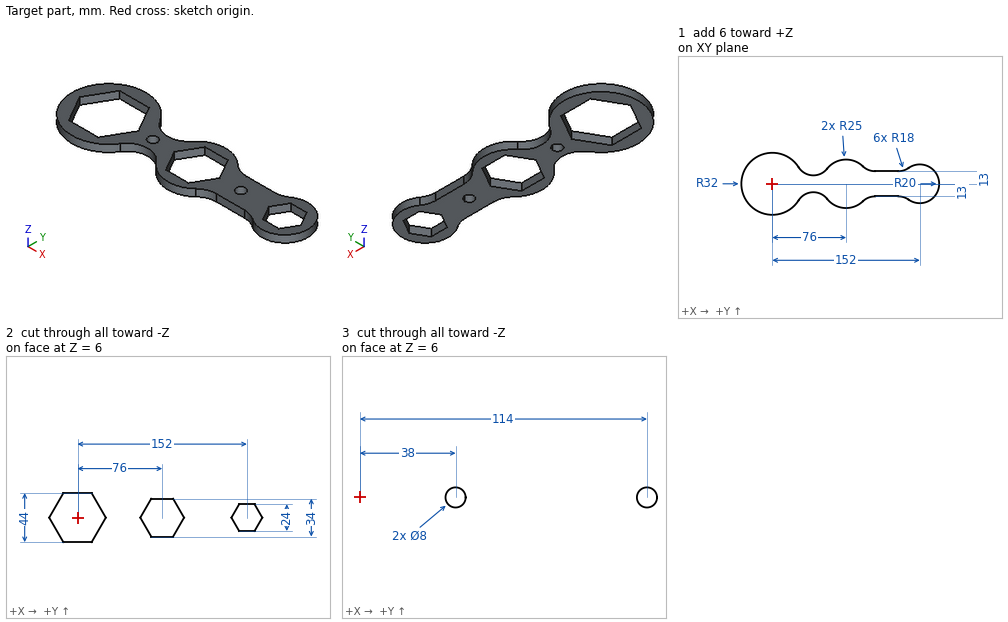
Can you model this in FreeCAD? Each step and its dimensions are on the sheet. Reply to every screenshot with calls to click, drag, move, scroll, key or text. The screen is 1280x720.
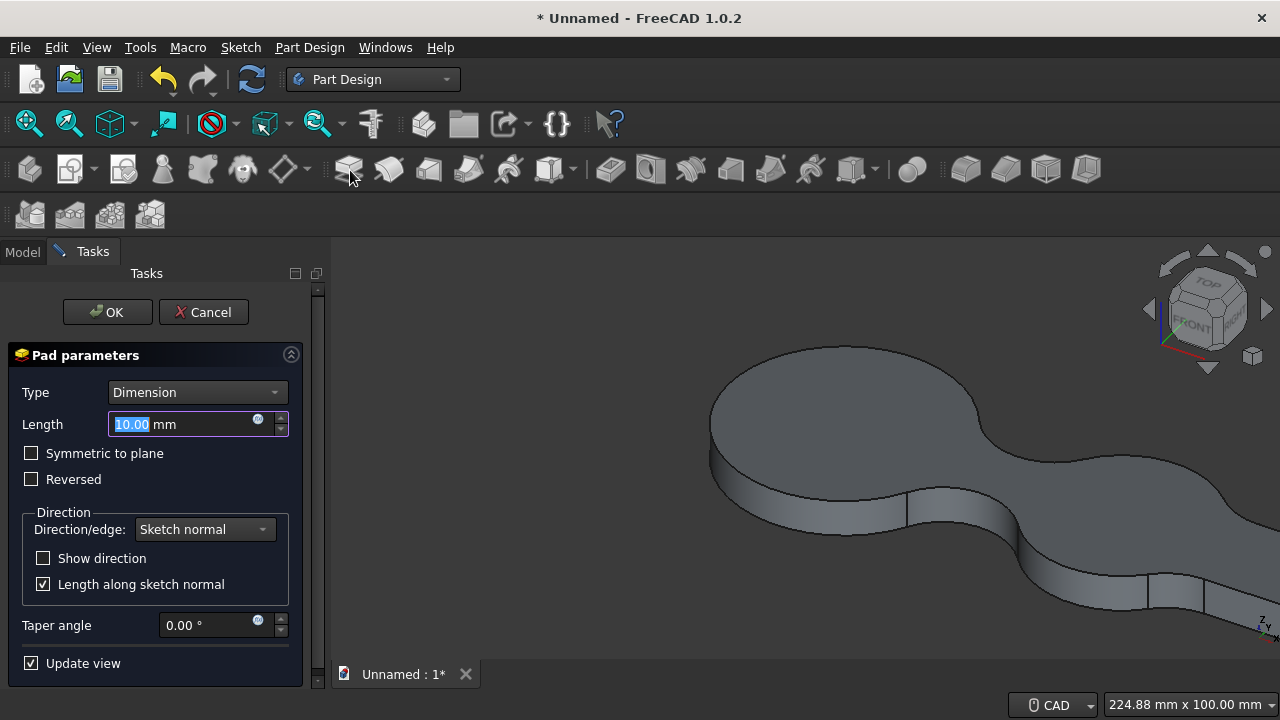
text(6)
key(Tab)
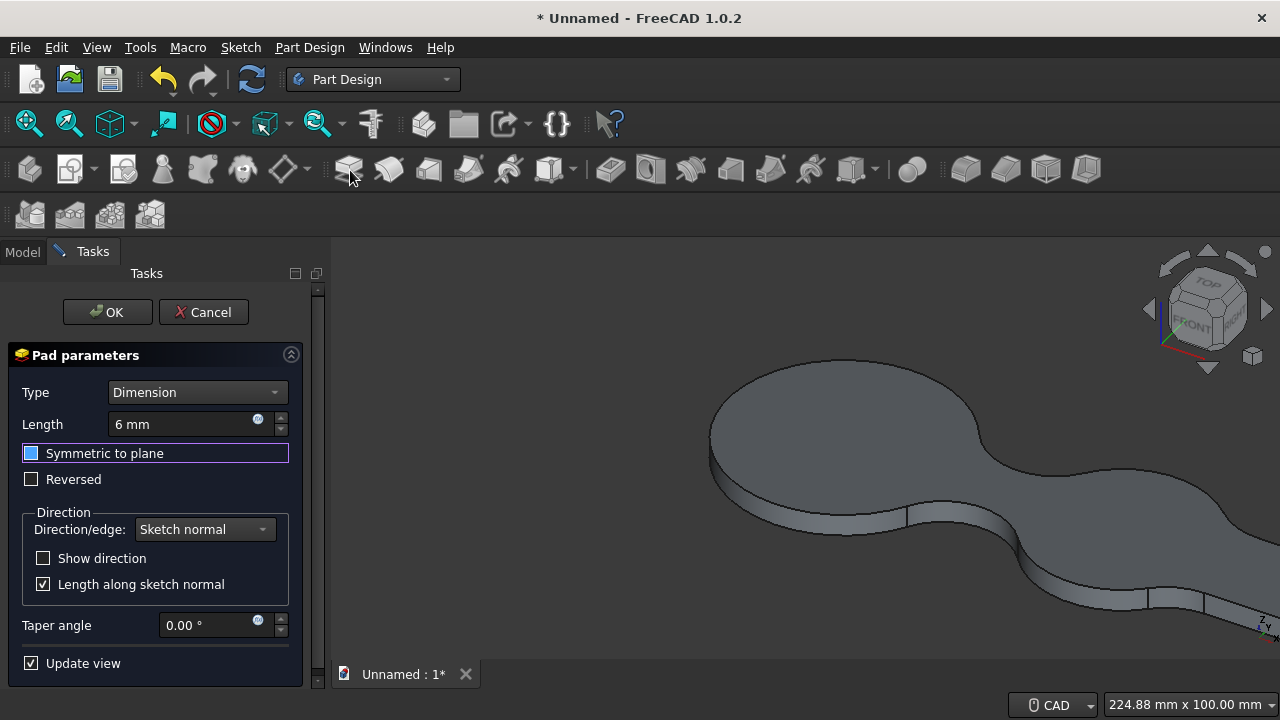
click(108, 312)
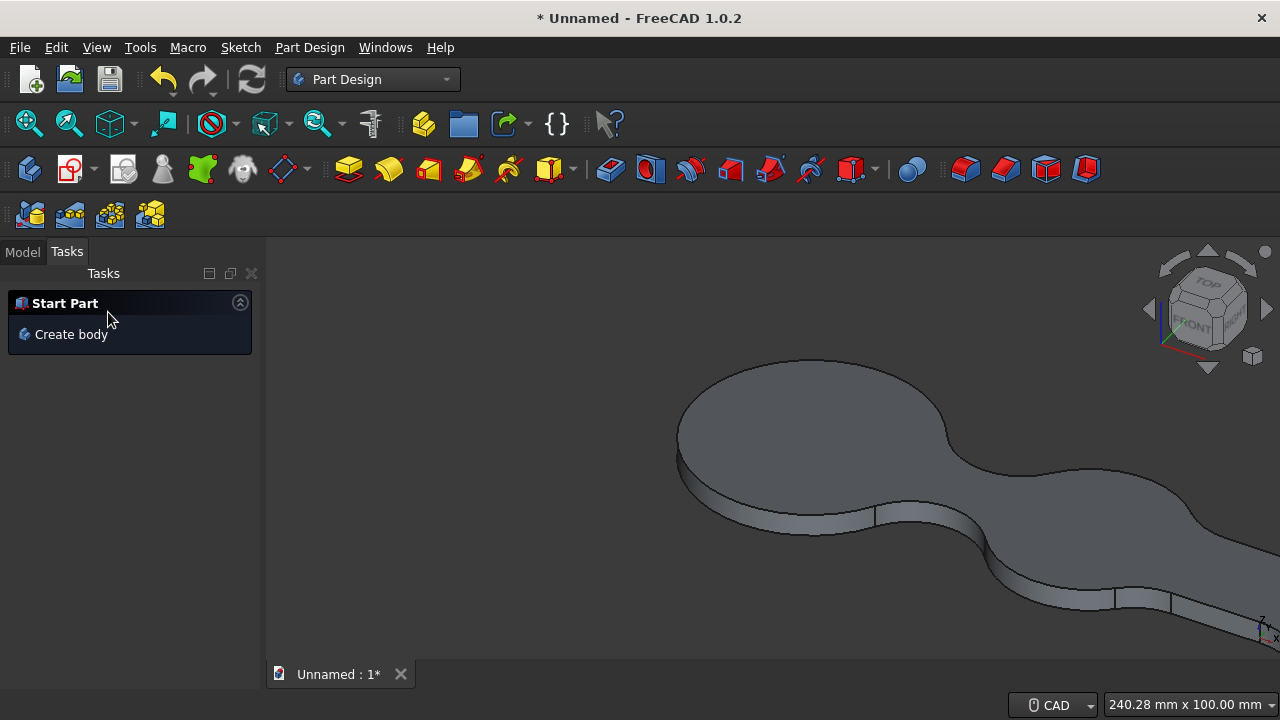
click(30, 124)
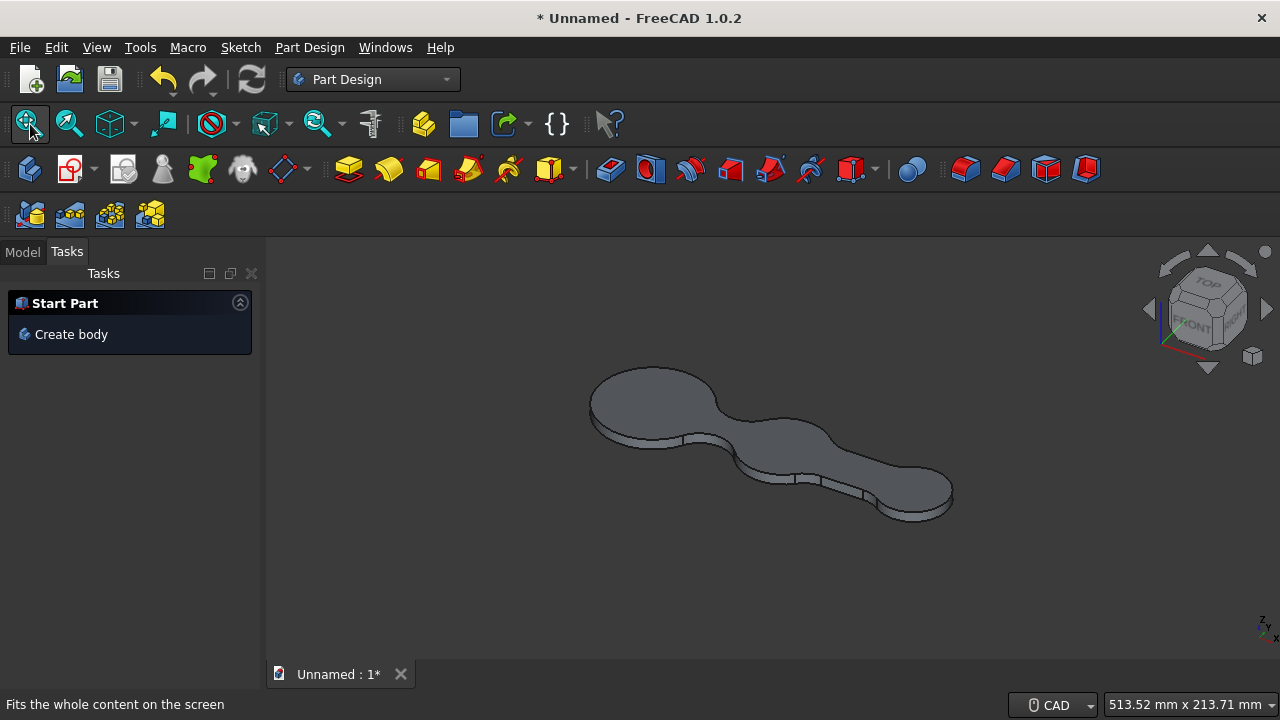
click(673, 409)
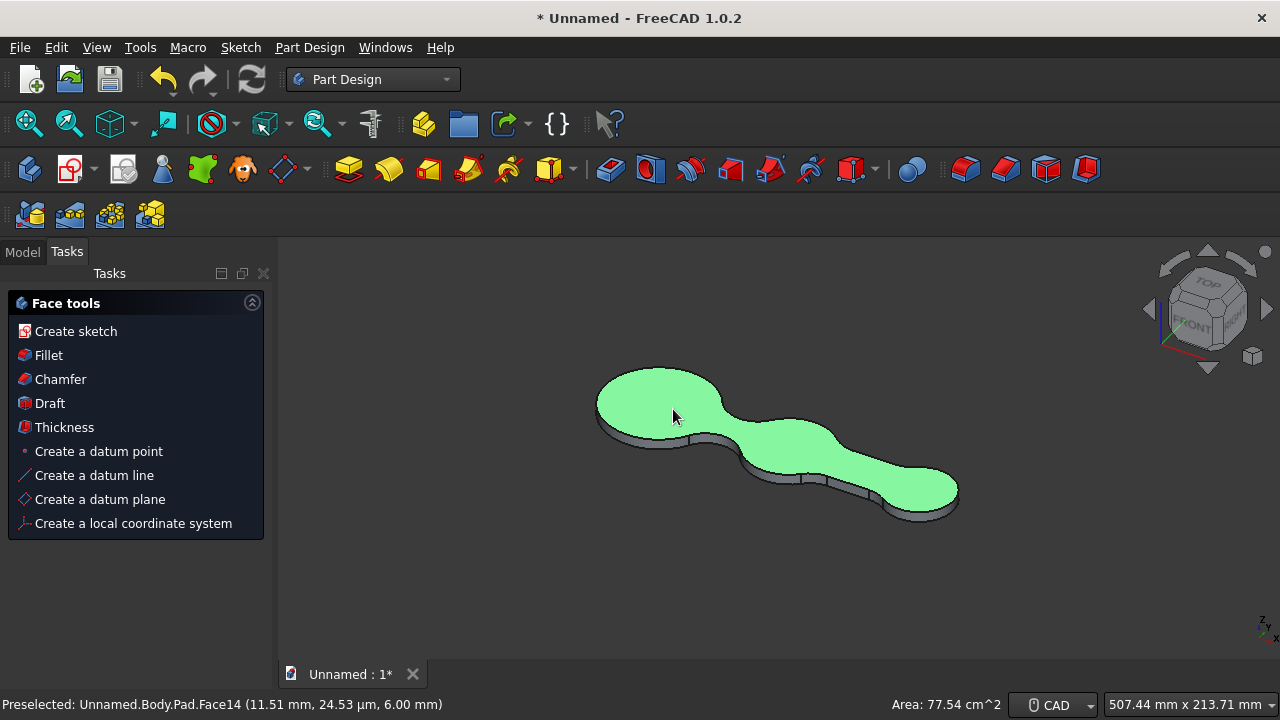
click(70, 170)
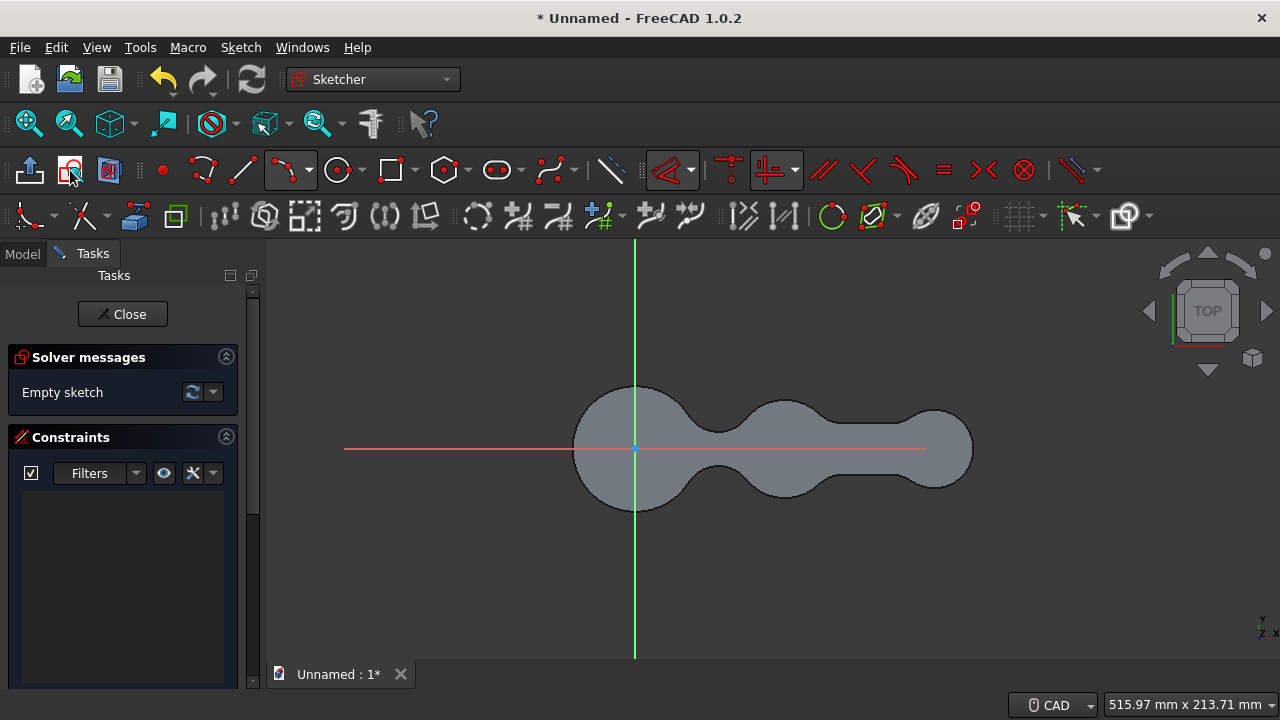
scroll(914, 449, up, 2)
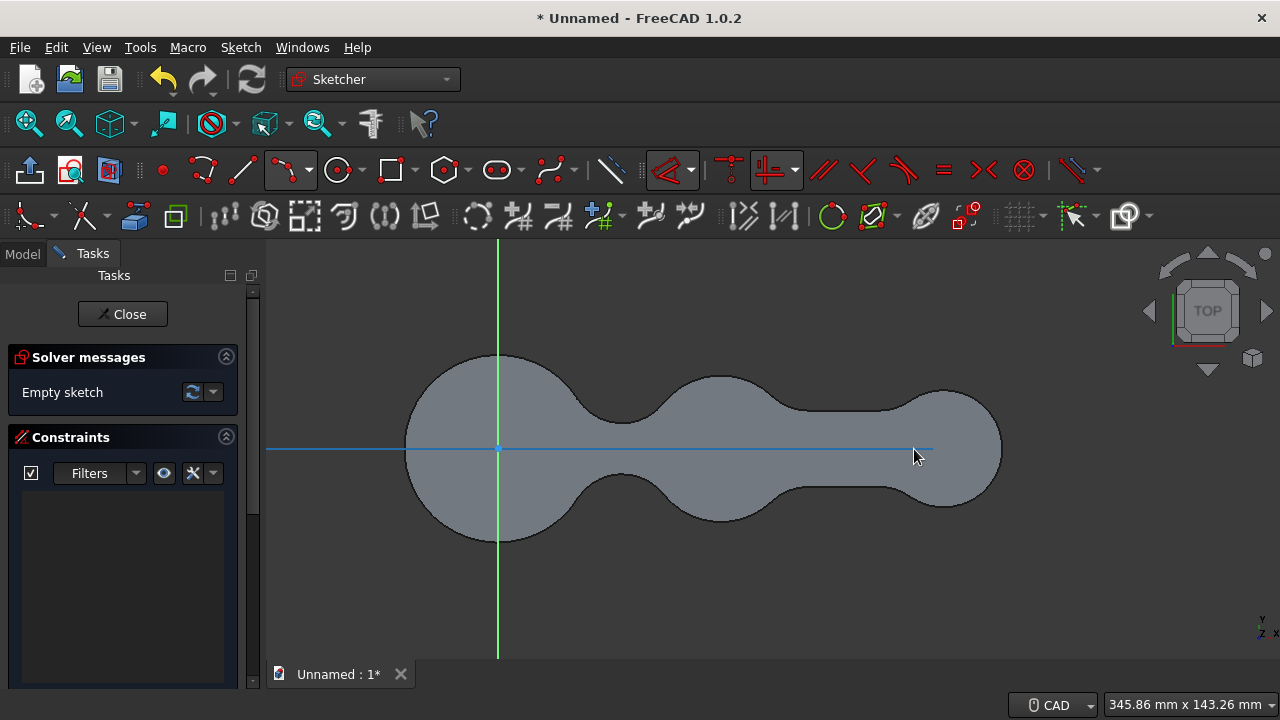
click(444, 170)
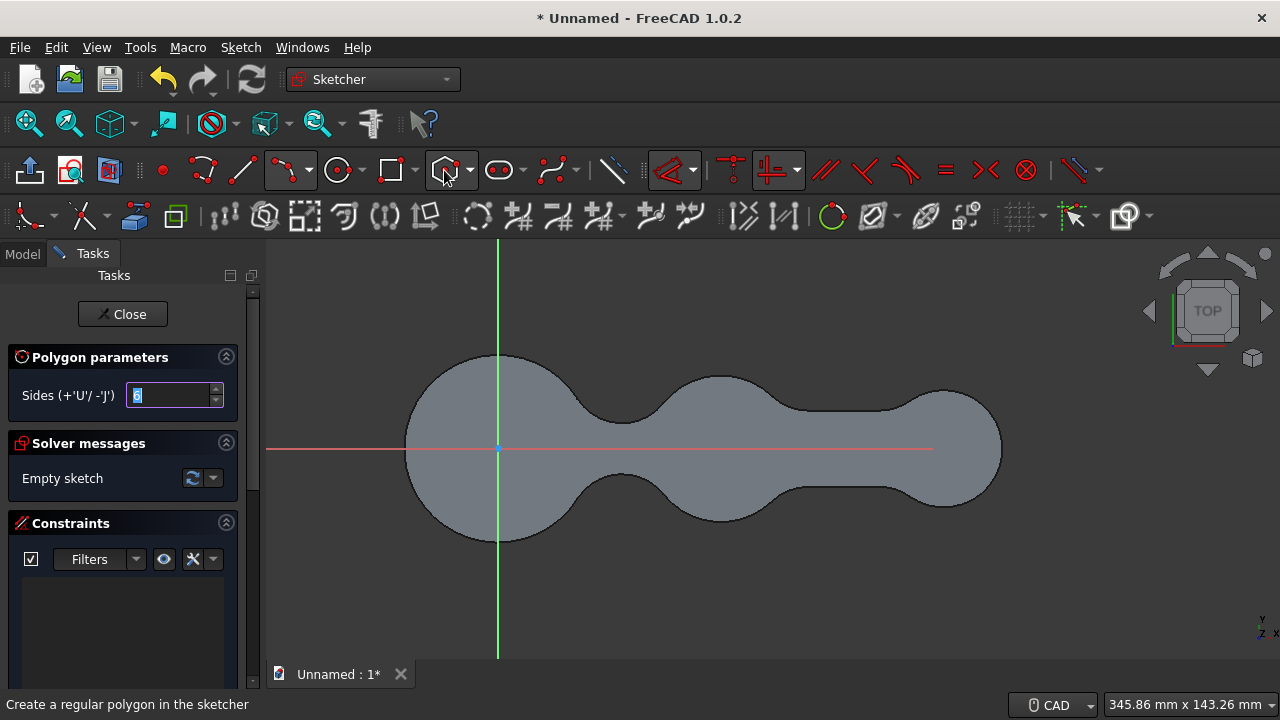
click(498, 449)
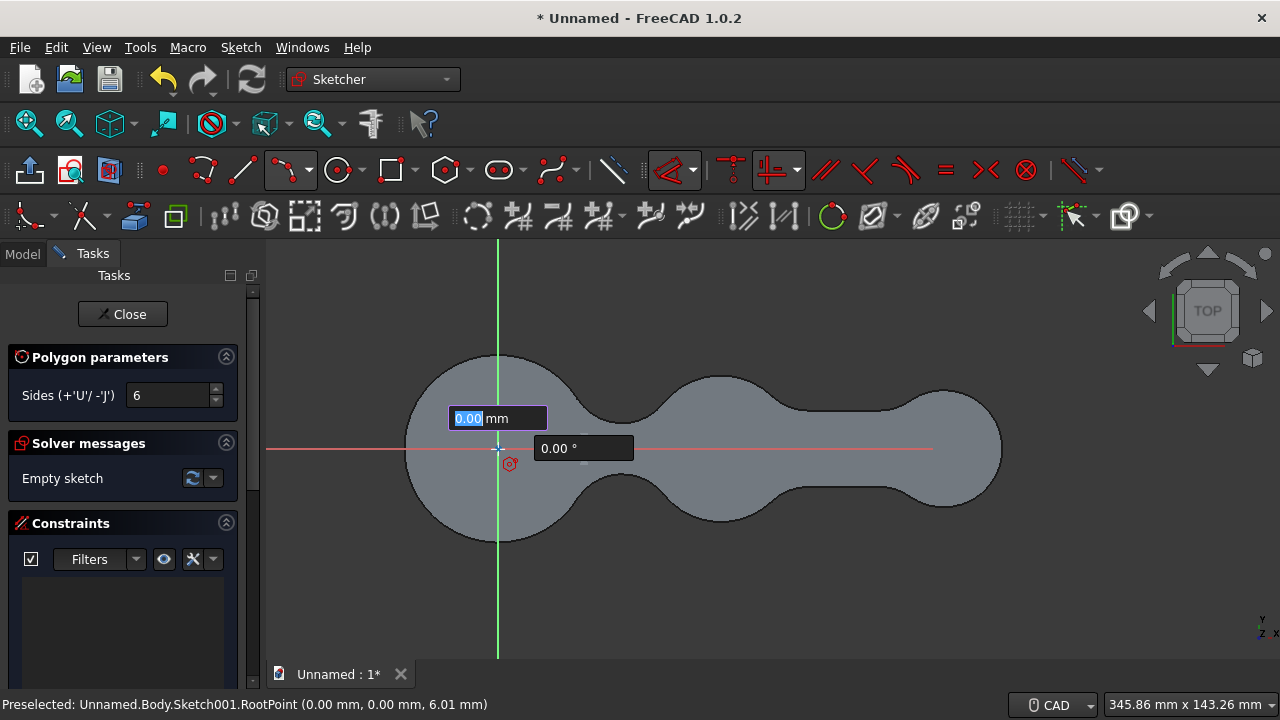
click(573, 449)
key(Escape)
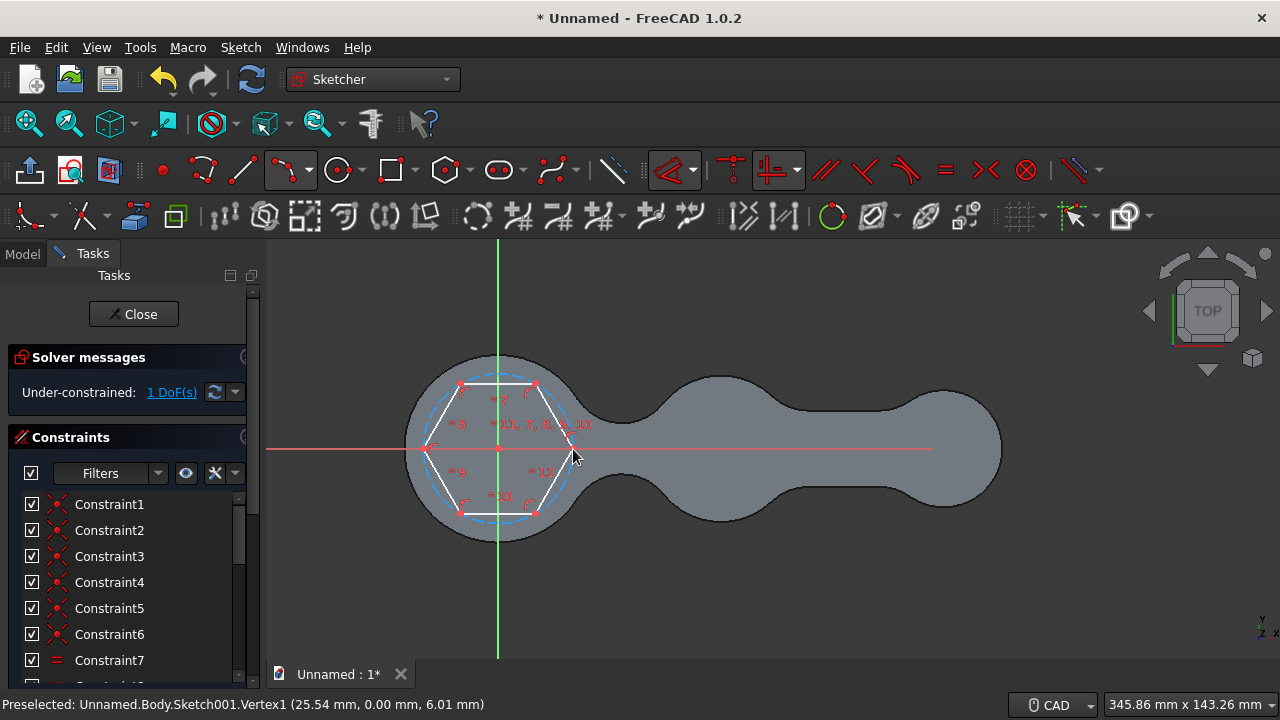
click(446, 170)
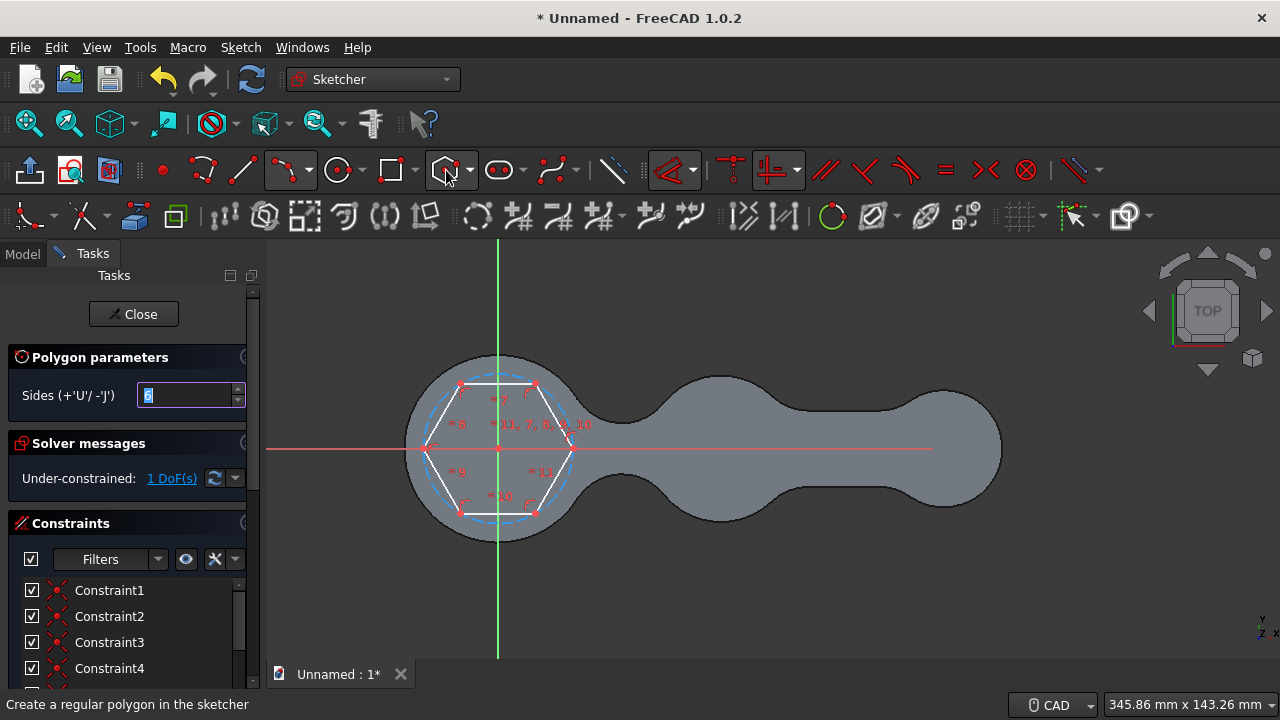
click(721, 449)